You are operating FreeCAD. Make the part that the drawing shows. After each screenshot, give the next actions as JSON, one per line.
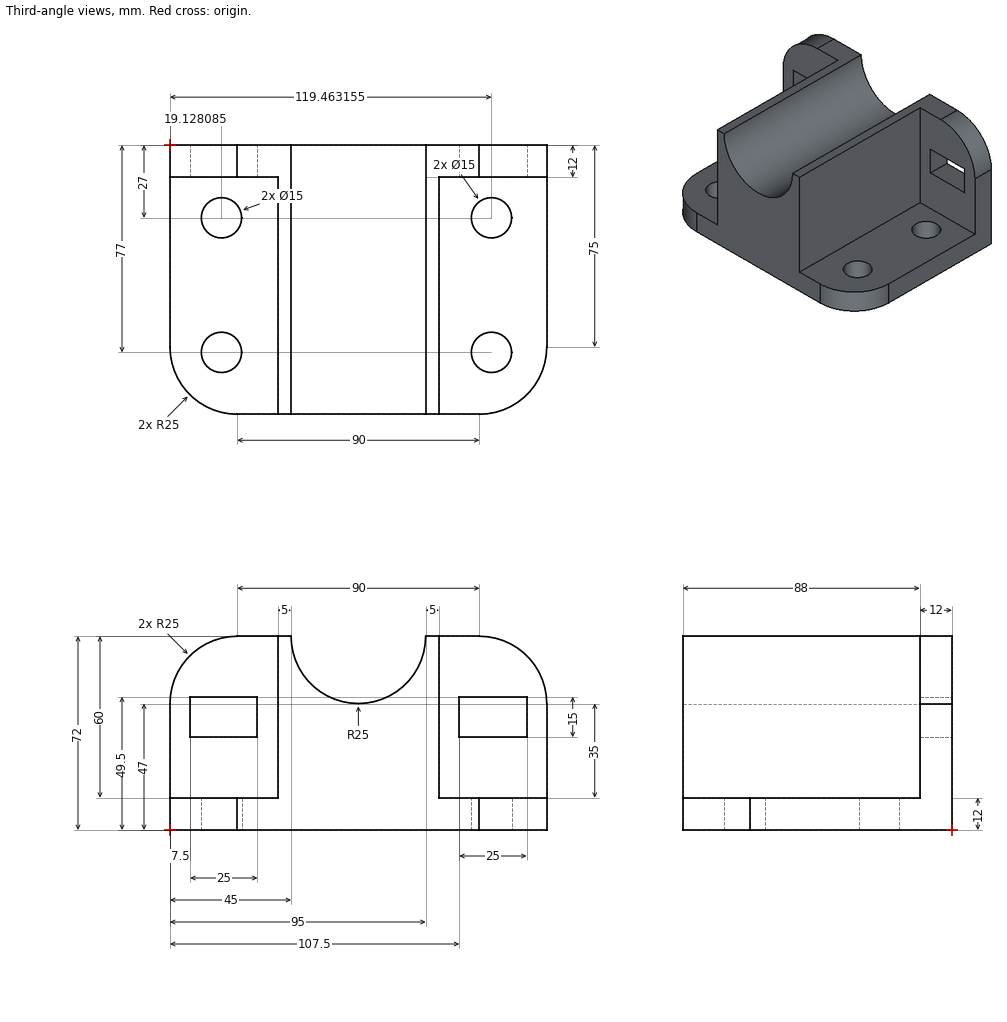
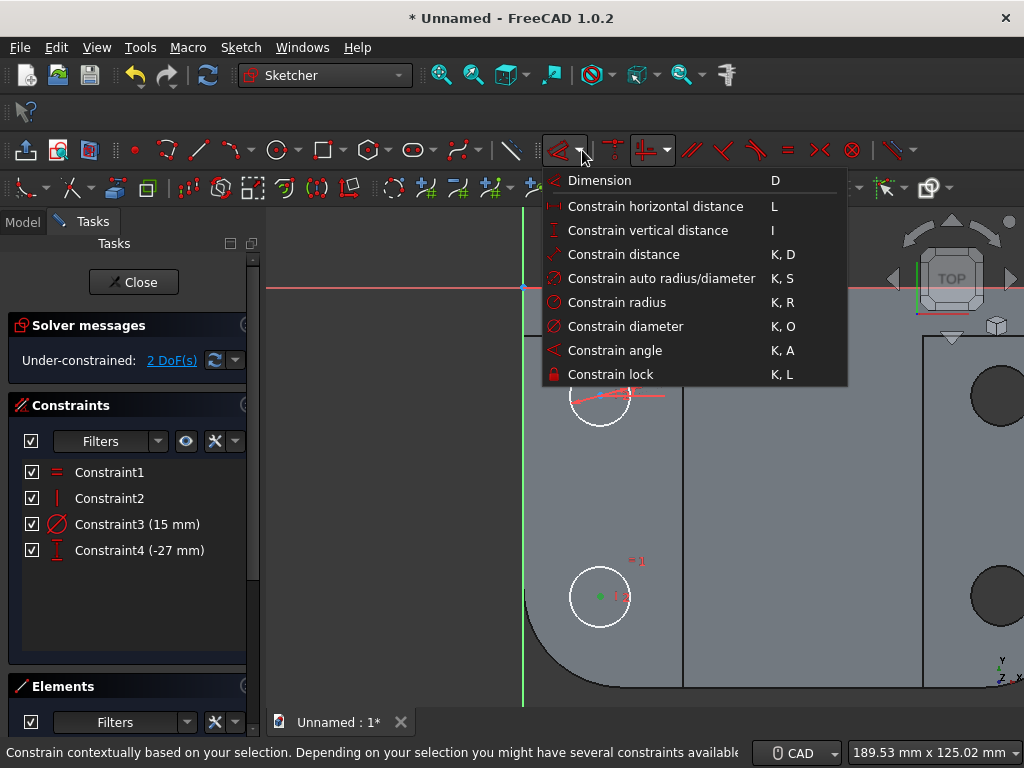
{"action": "left_click", "coordinate": [695, 230]}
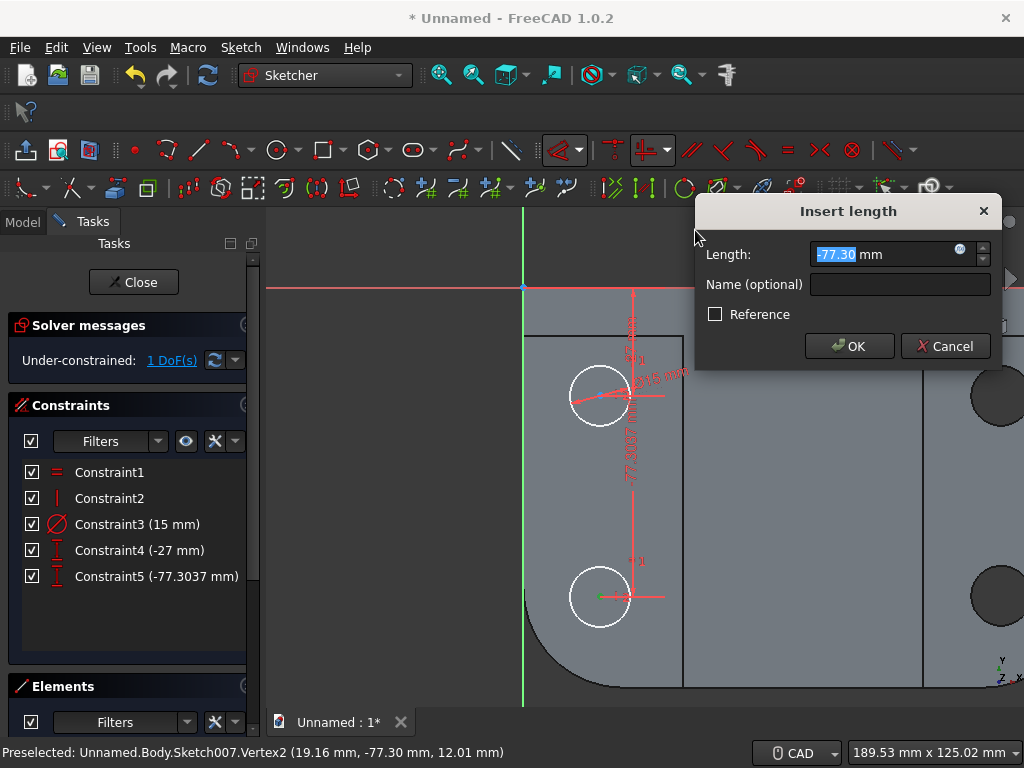
{"action": "type", "text": "-77"}
{"action": "key", "text": "Return"}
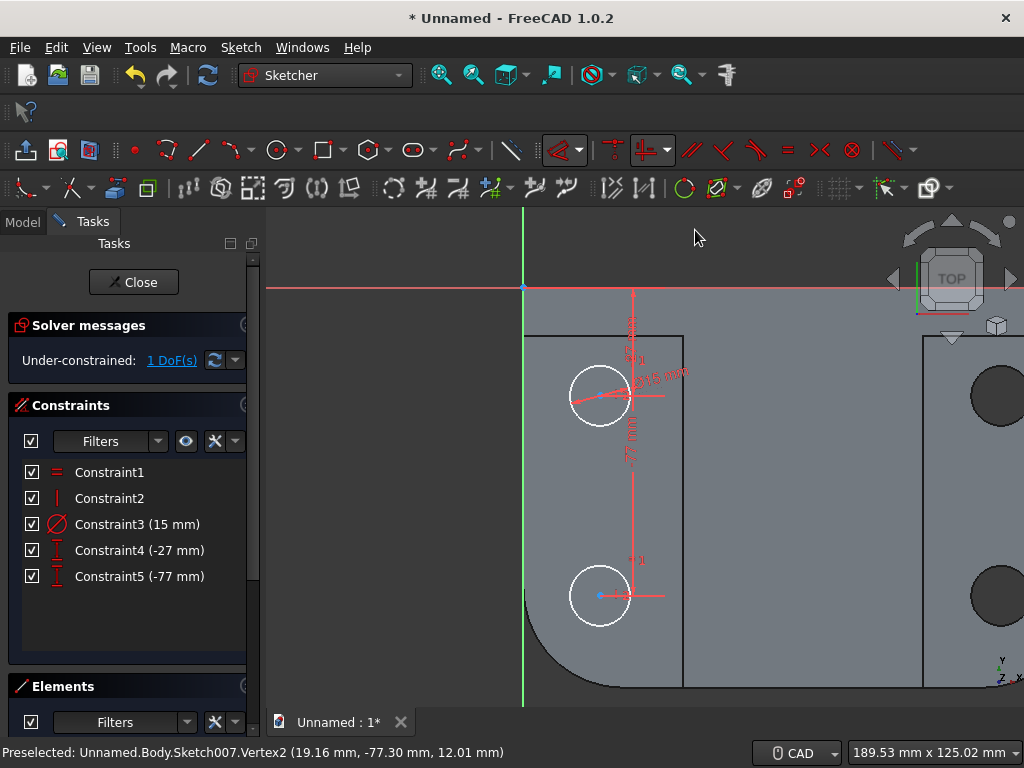
{"action": "left_click", "coordinate": [600, 396]}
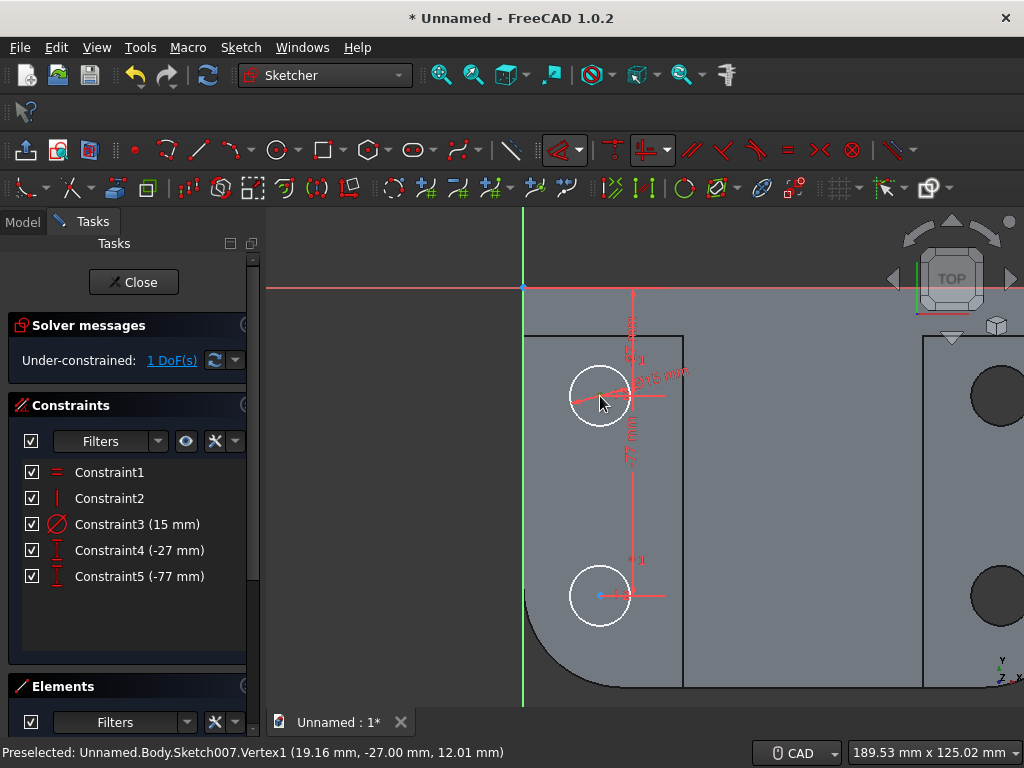
{"action": "key", "text": "l"}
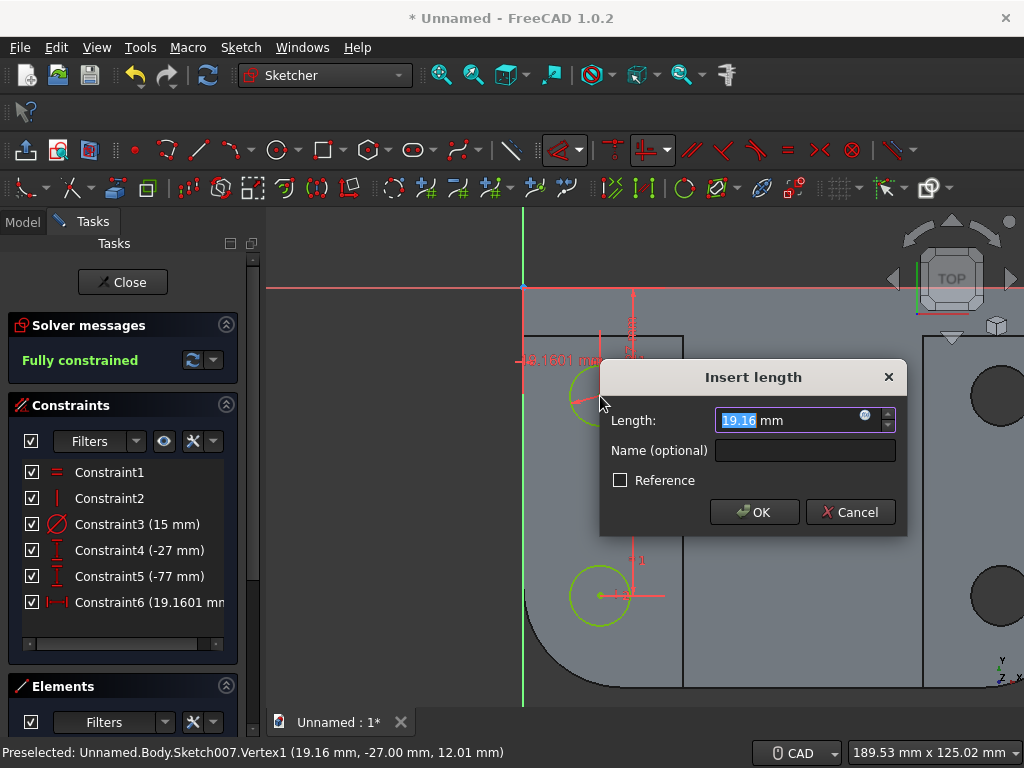
{"action": "type", "text": "19.128085"}
{"action": "key", "text": "Return"}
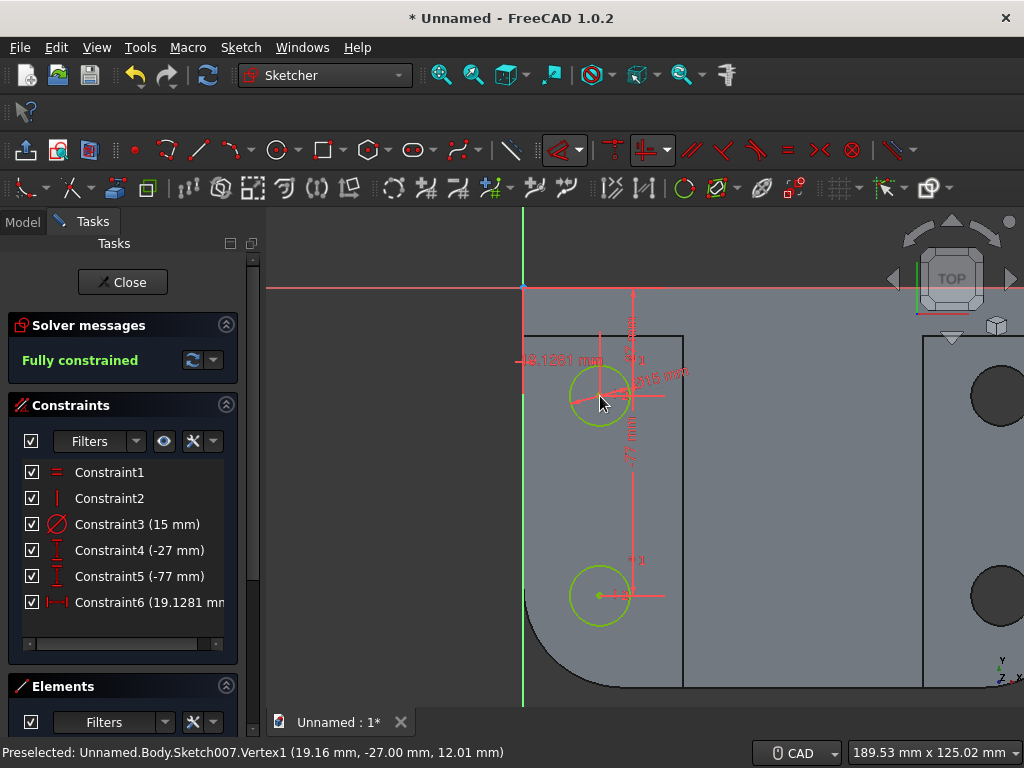
{"action": "left_click", "coordinate": [123, 282]}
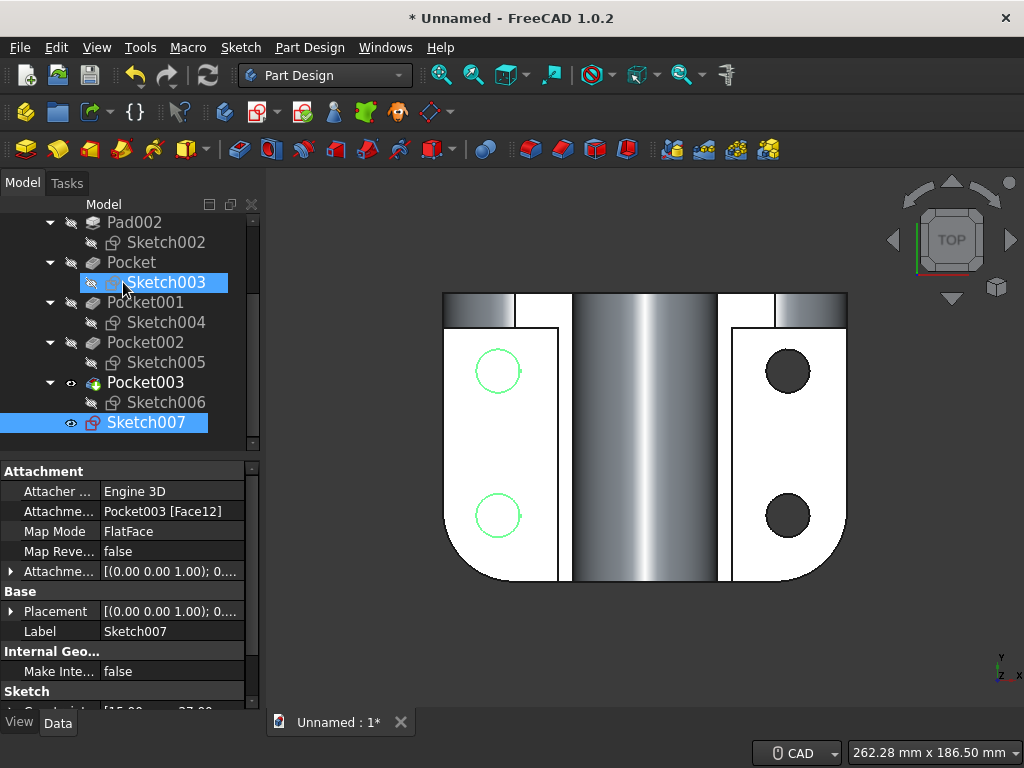
{"action": "left_click", "coordinate": [240, 150]}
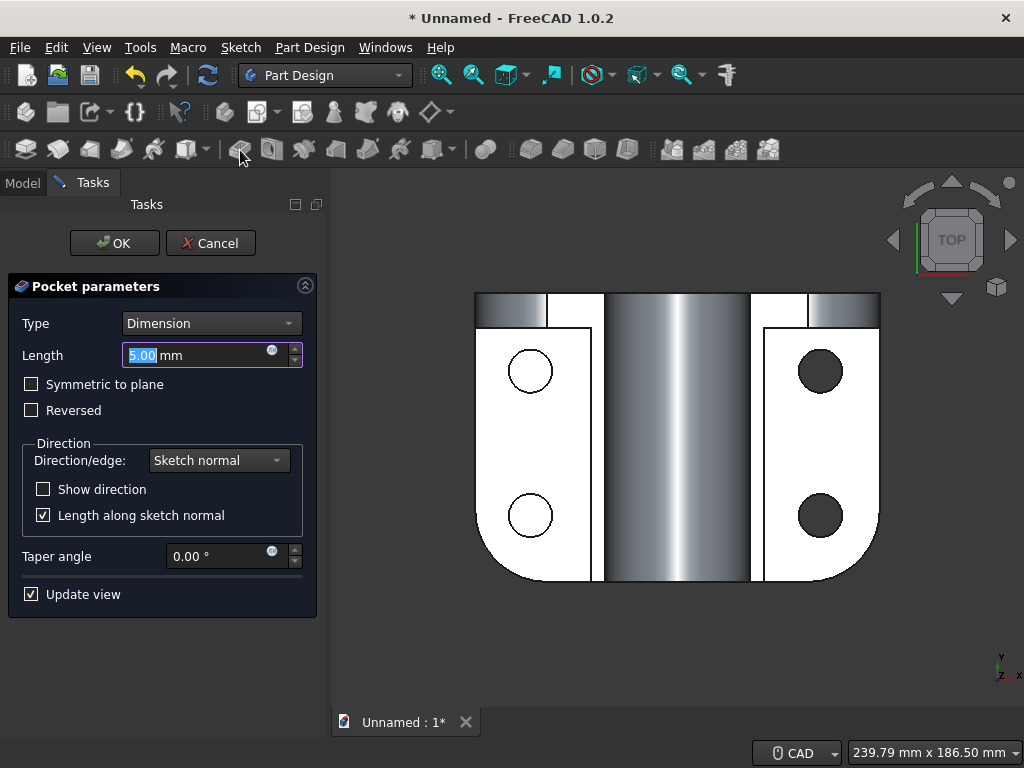
{"action": "type", "text": "12"}
{"action": "key", "text": "Tab"}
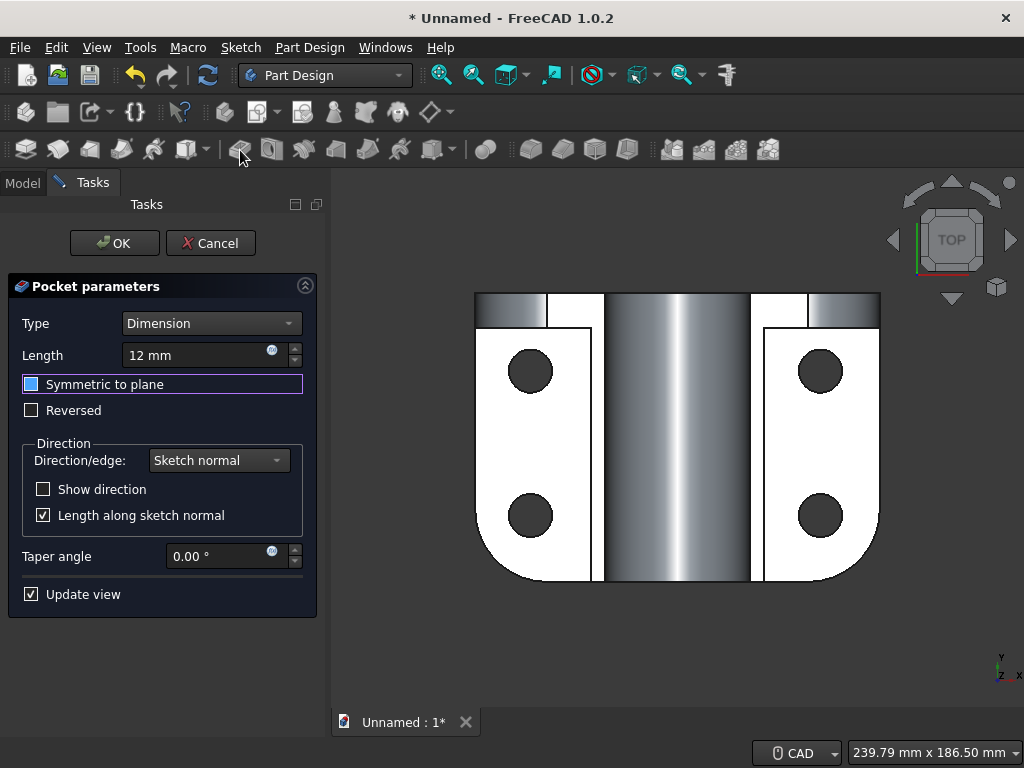
{"action": "left_click", "coordinate": [115, 243]}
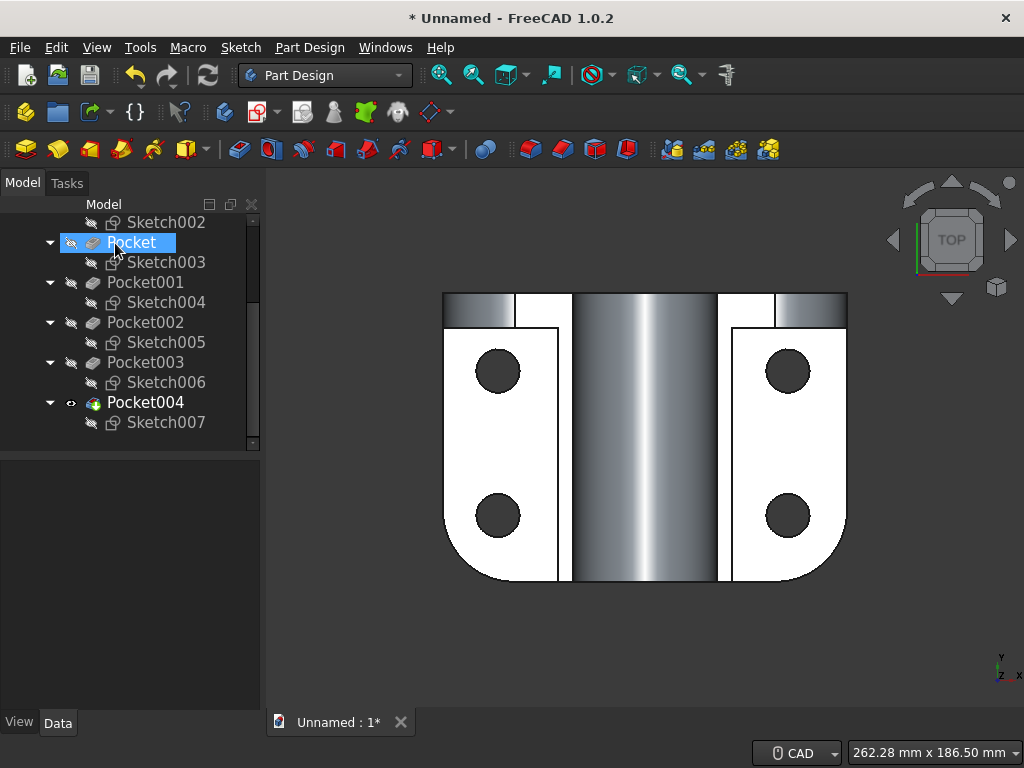
{"action": "key", "text": "0"}